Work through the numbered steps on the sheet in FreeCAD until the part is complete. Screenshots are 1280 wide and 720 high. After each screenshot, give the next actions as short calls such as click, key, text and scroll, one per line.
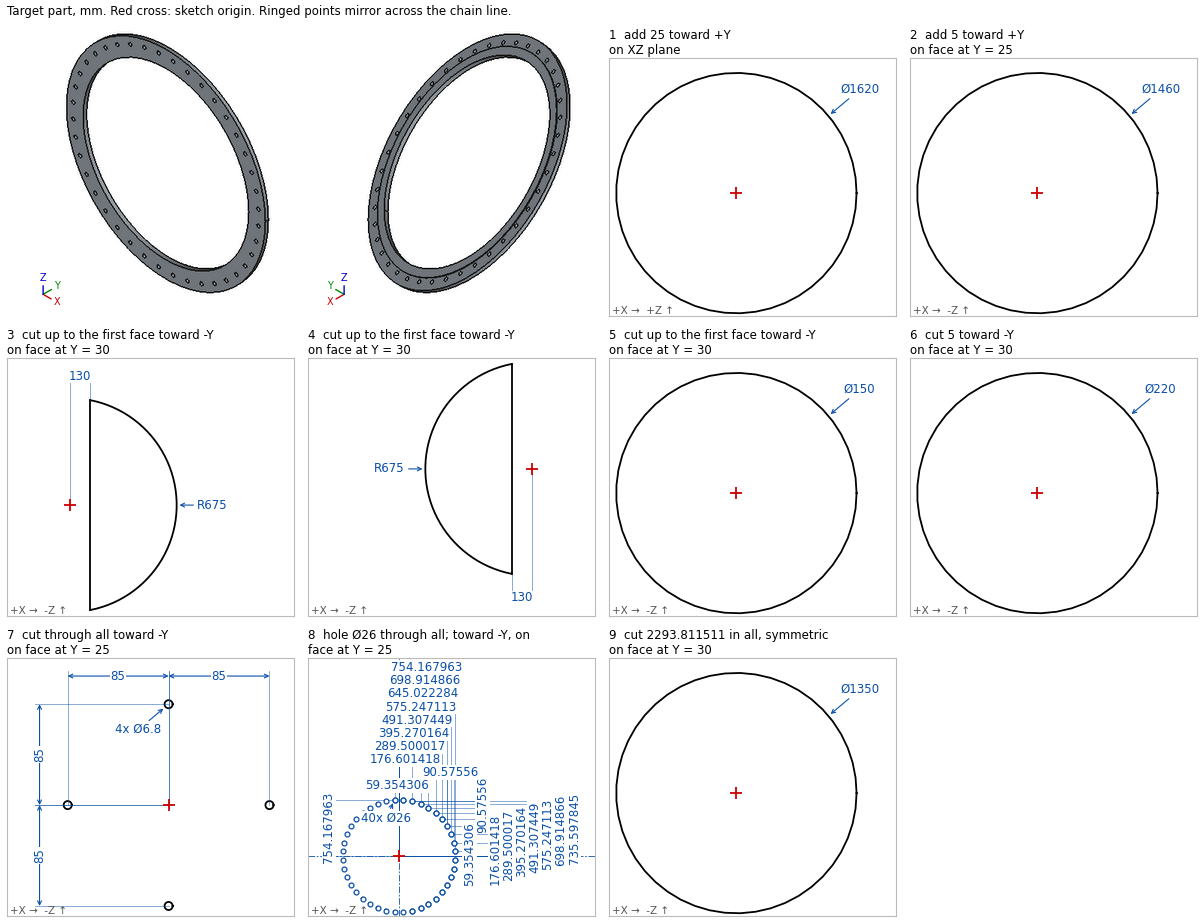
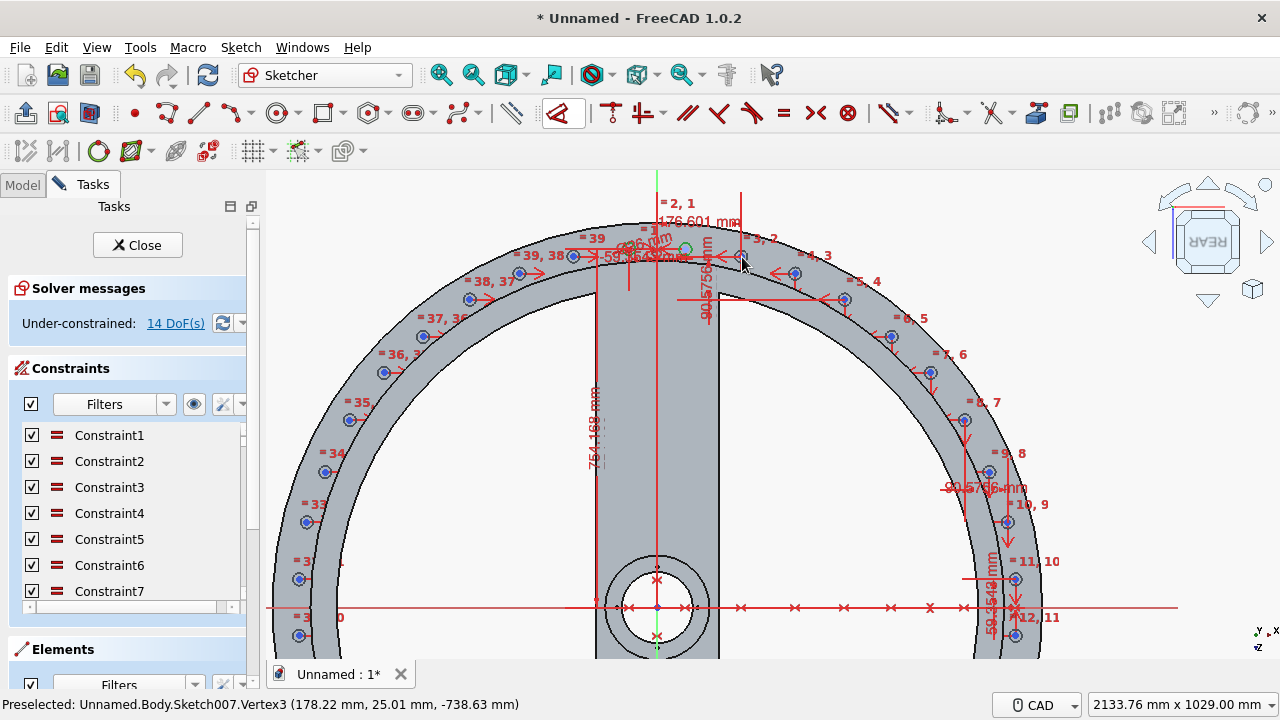
click(741, 257)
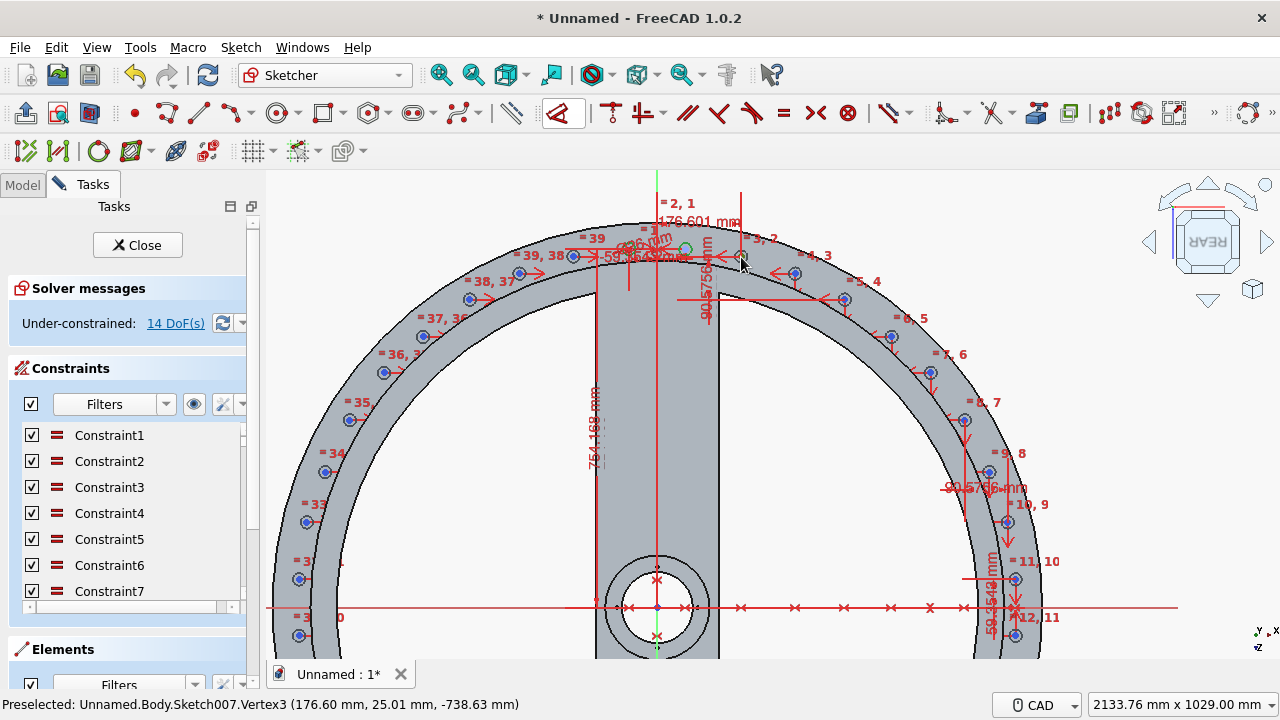
click(580, 114)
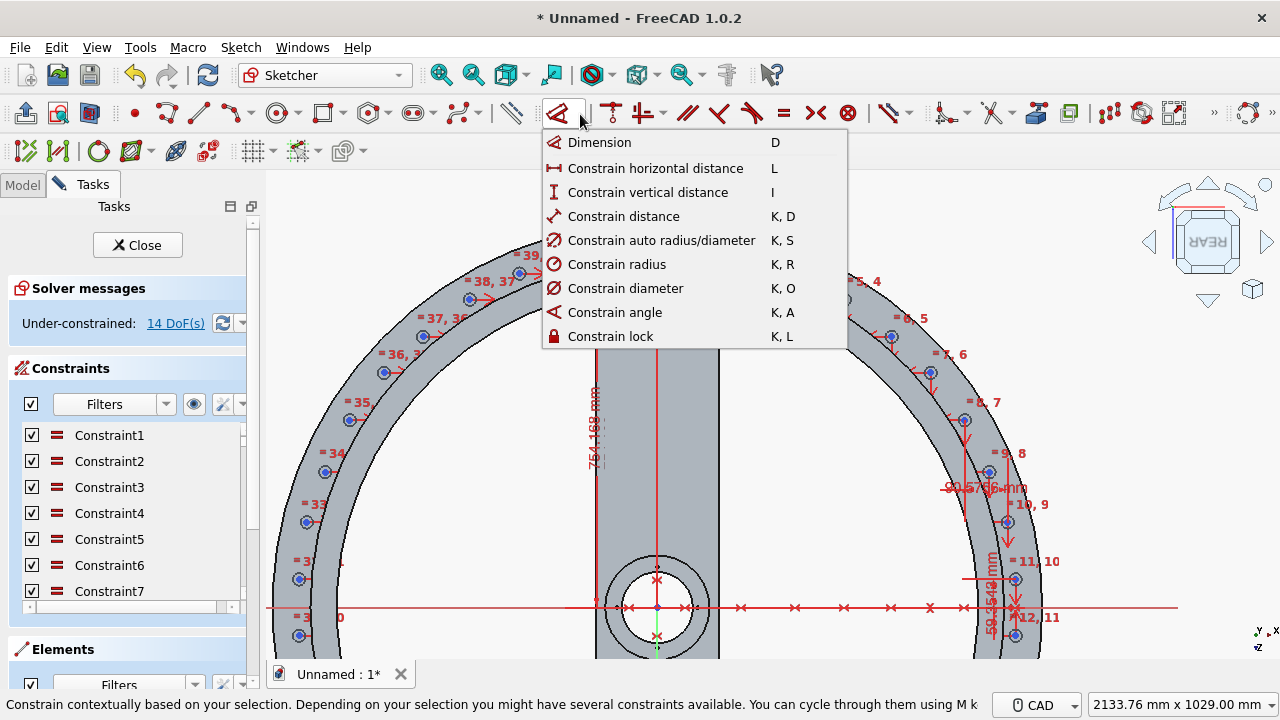
click(695, 192)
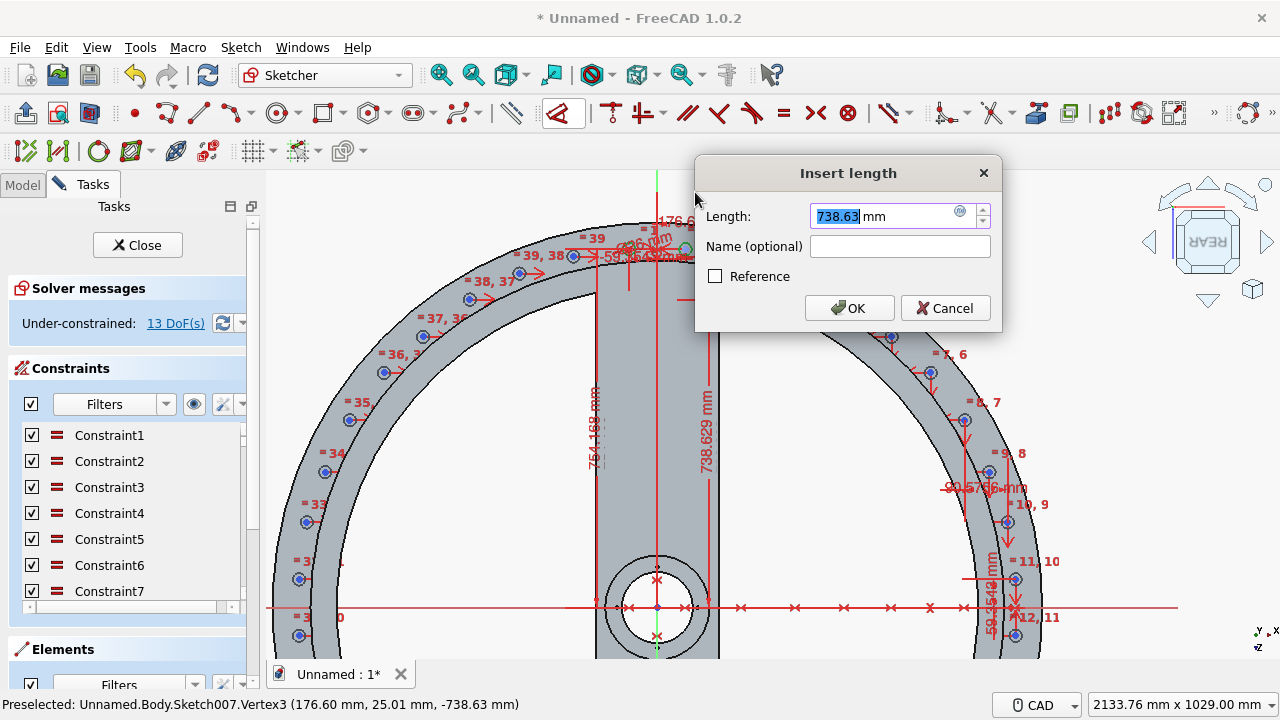
text(735.597845)
key(Return)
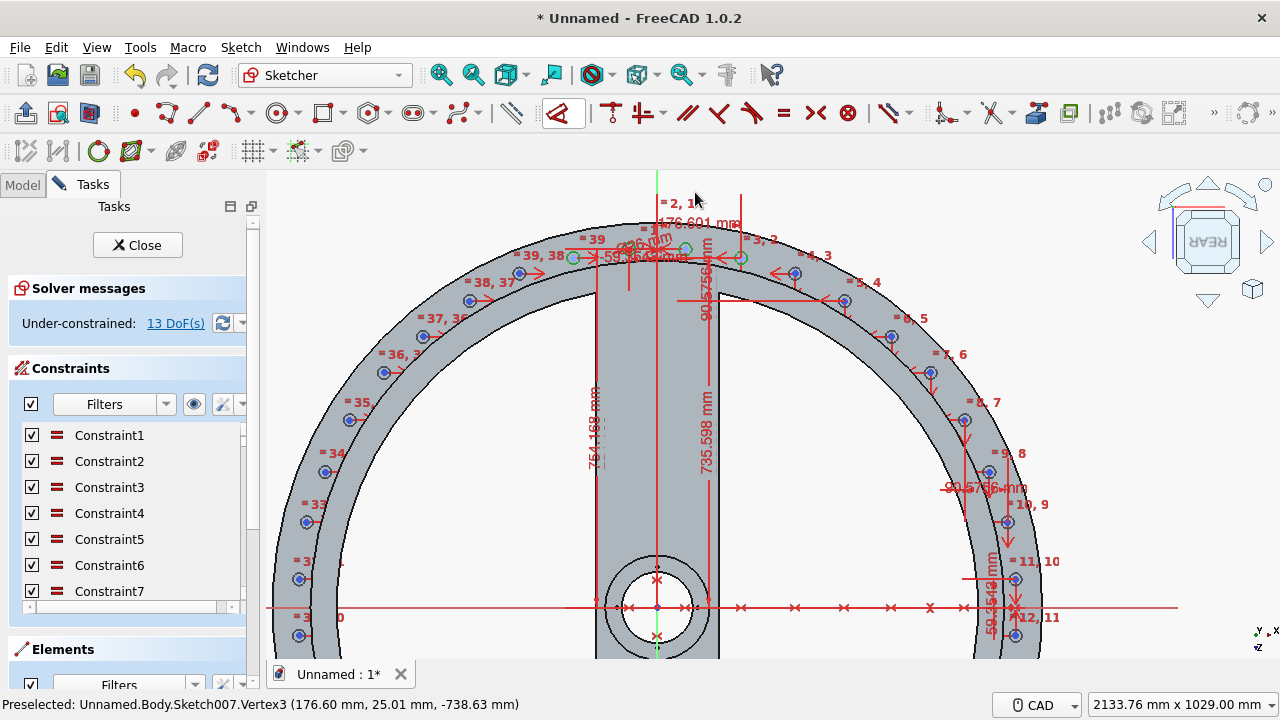
click(795, 274)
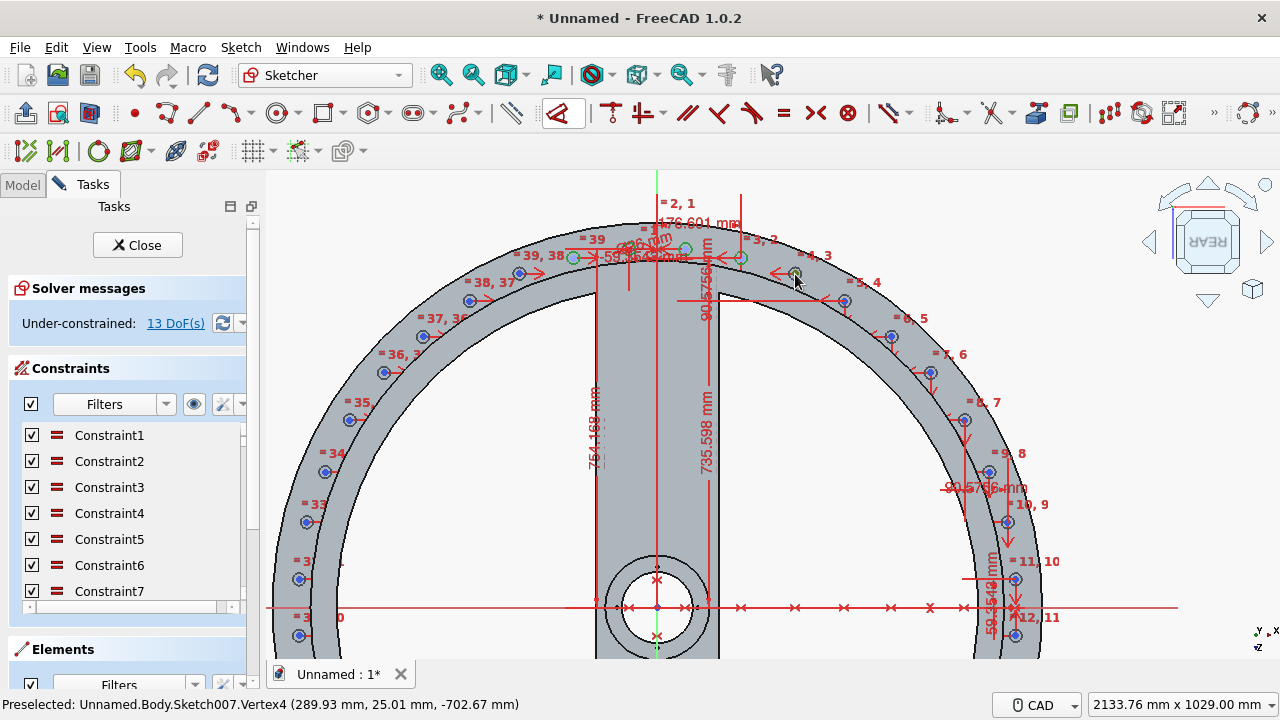
key(l)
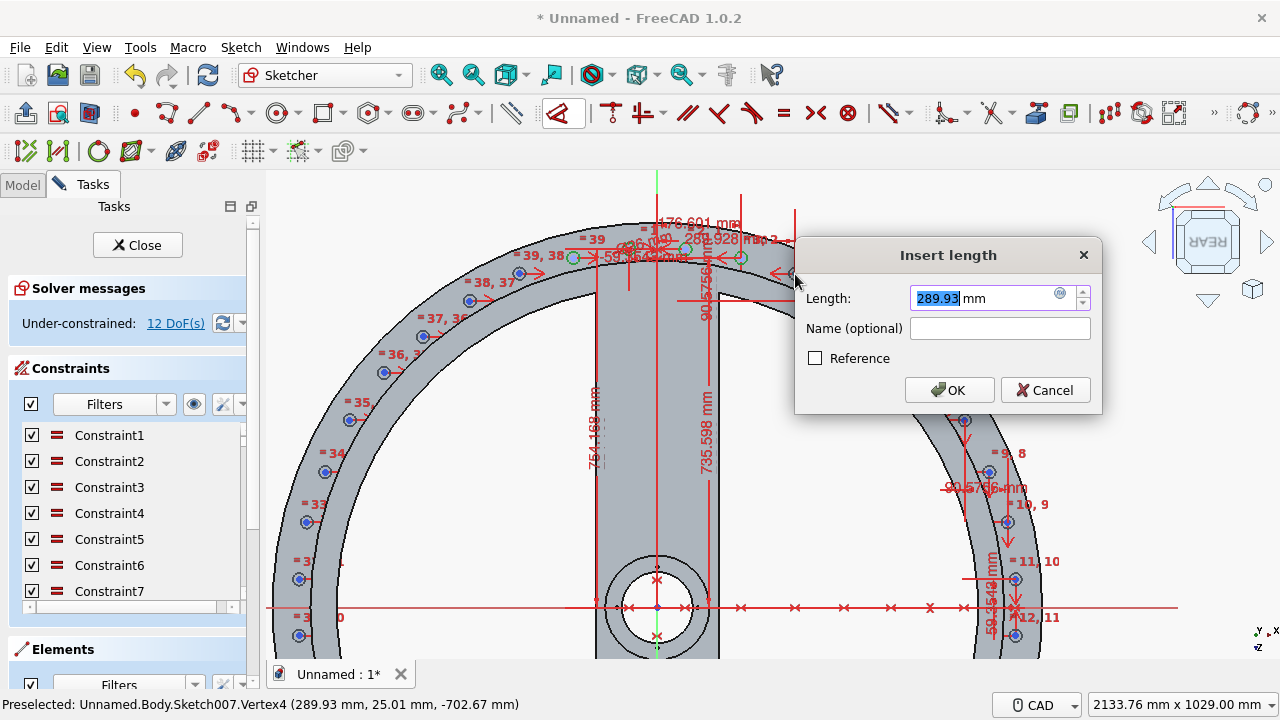
text(289.500017)
key(Return)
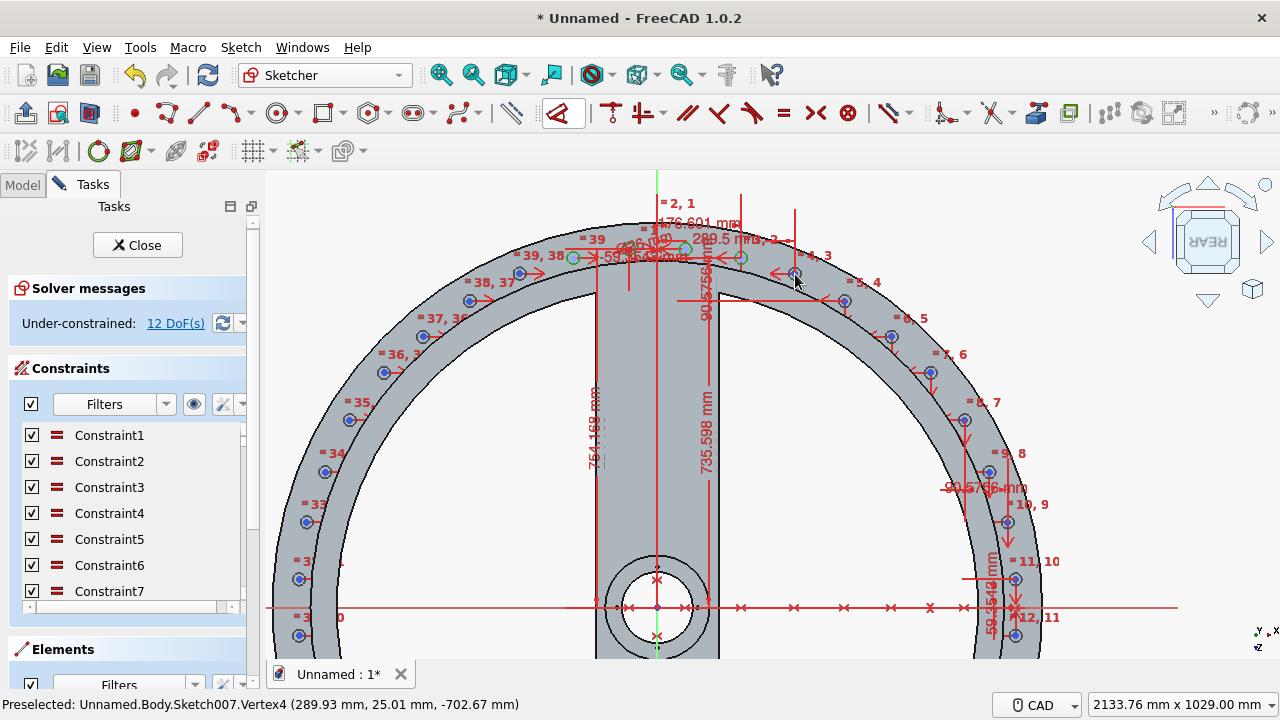
click(795, 274)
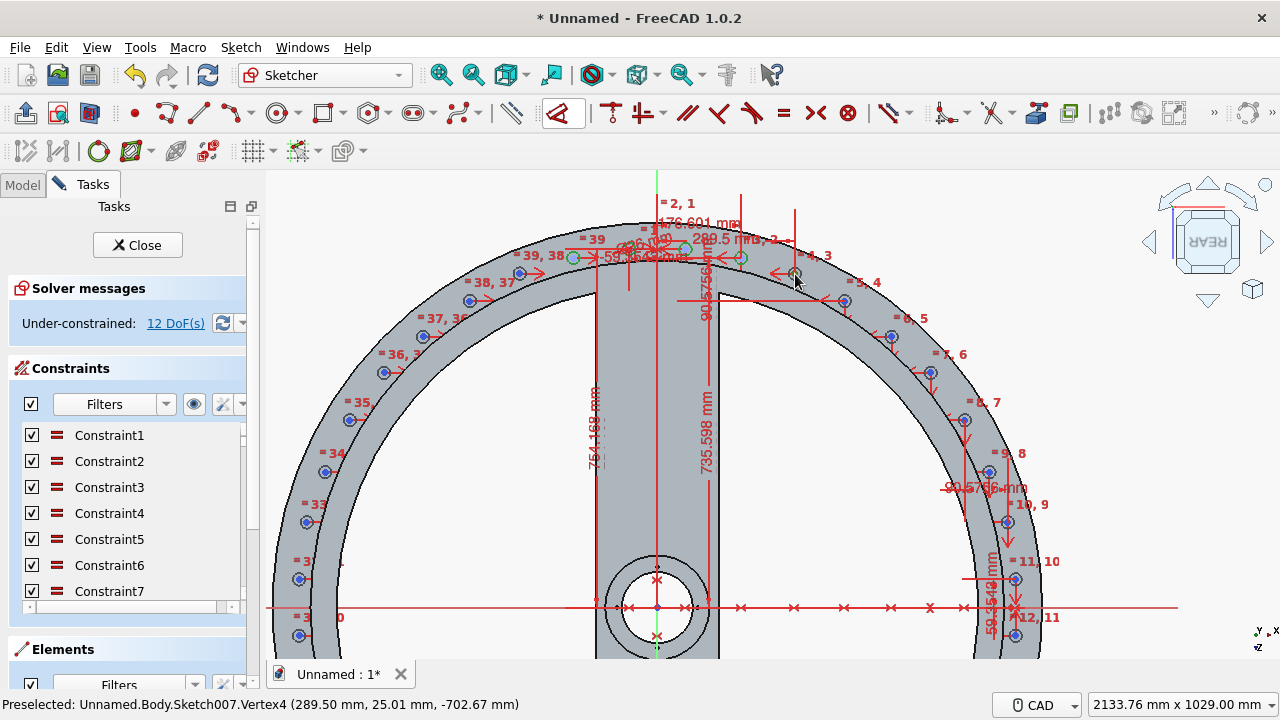
key(i)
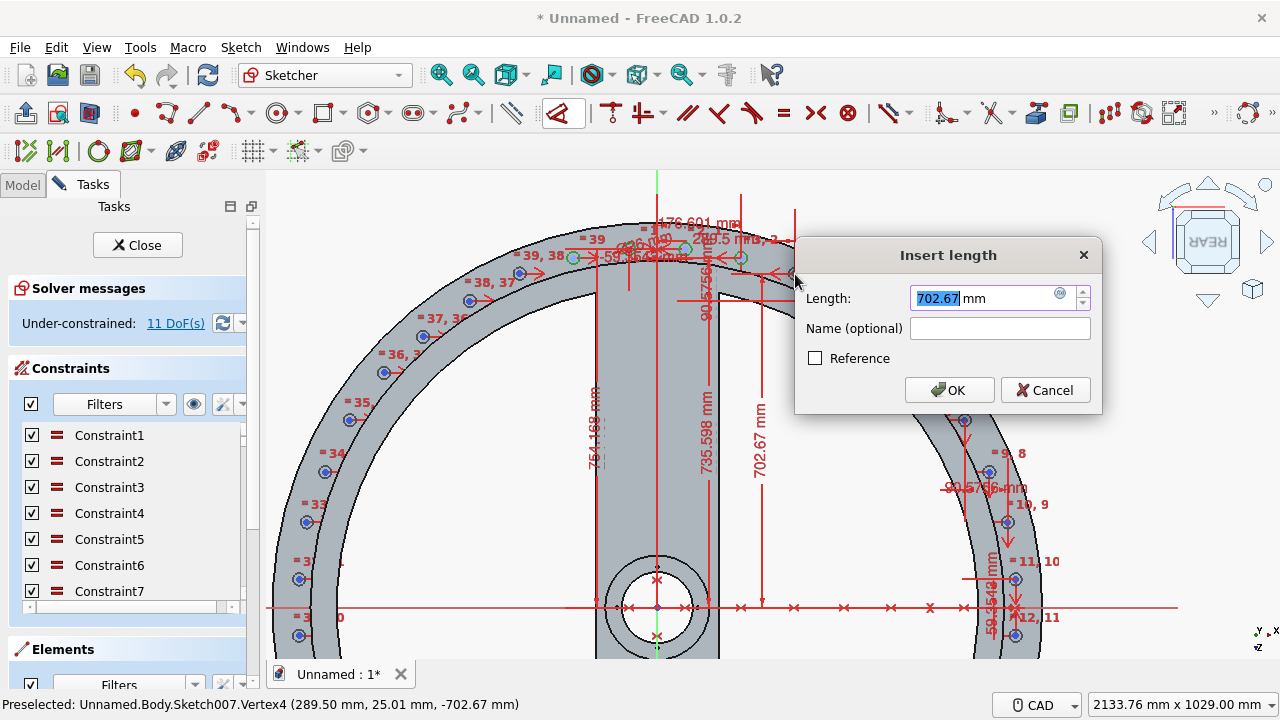
text(698.914866)
key(Return)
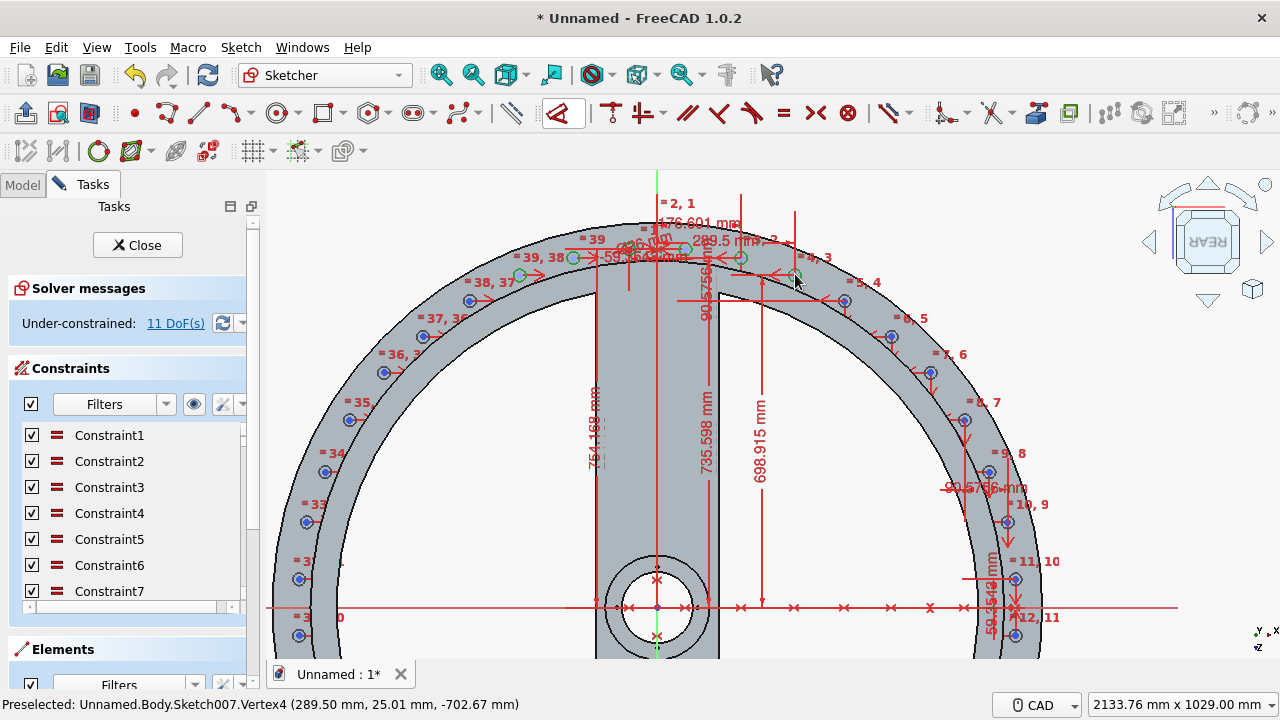
click(845, 301)